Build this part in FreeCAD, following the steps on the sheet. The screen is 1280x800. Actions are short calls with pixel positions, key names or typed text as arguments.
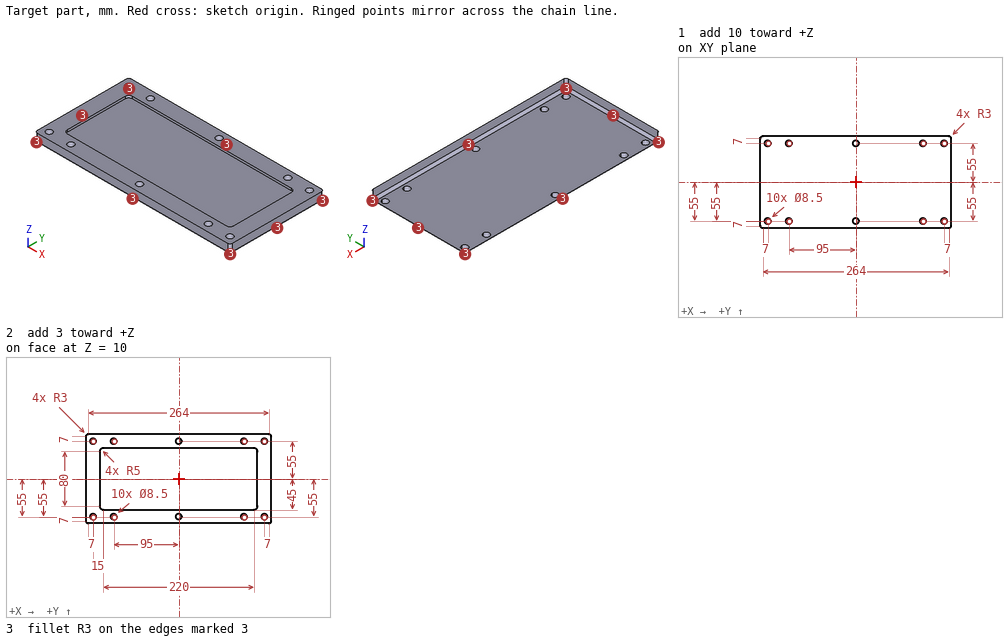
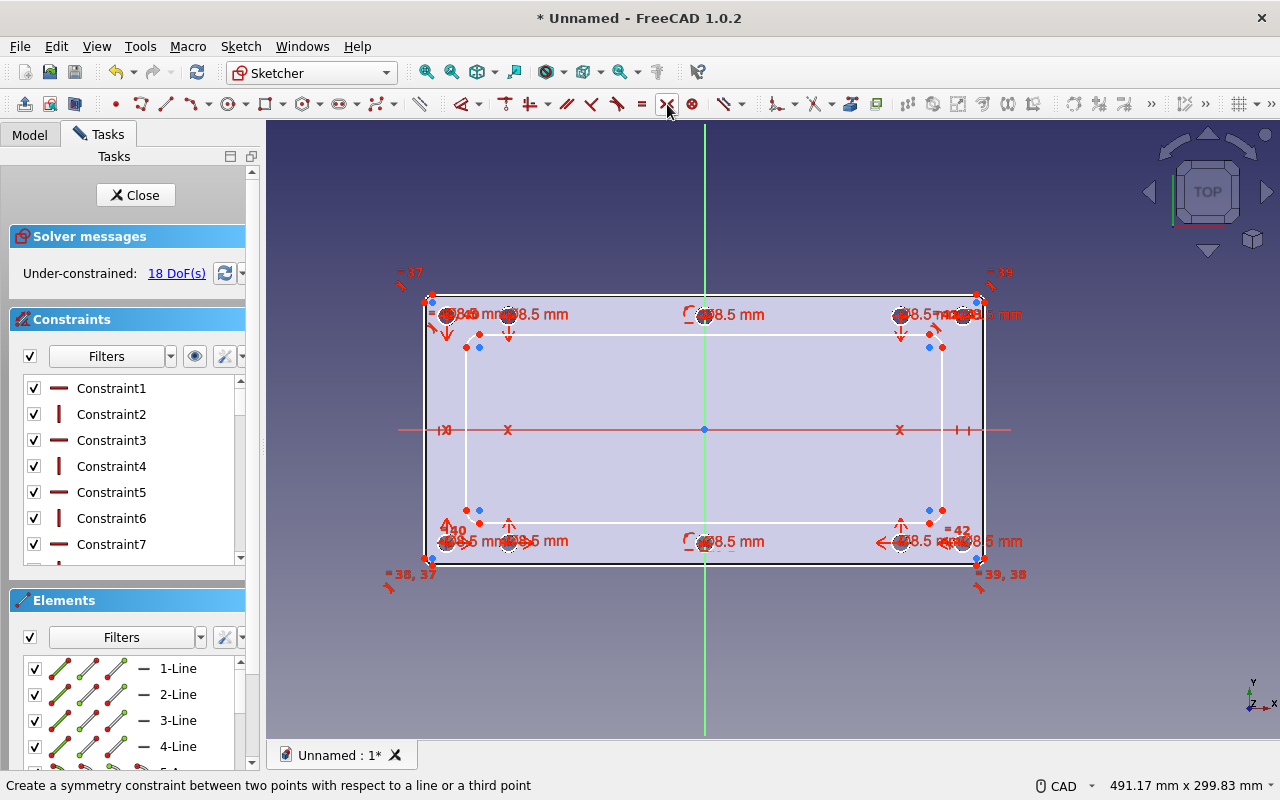
scroll(963, 543, up, 4)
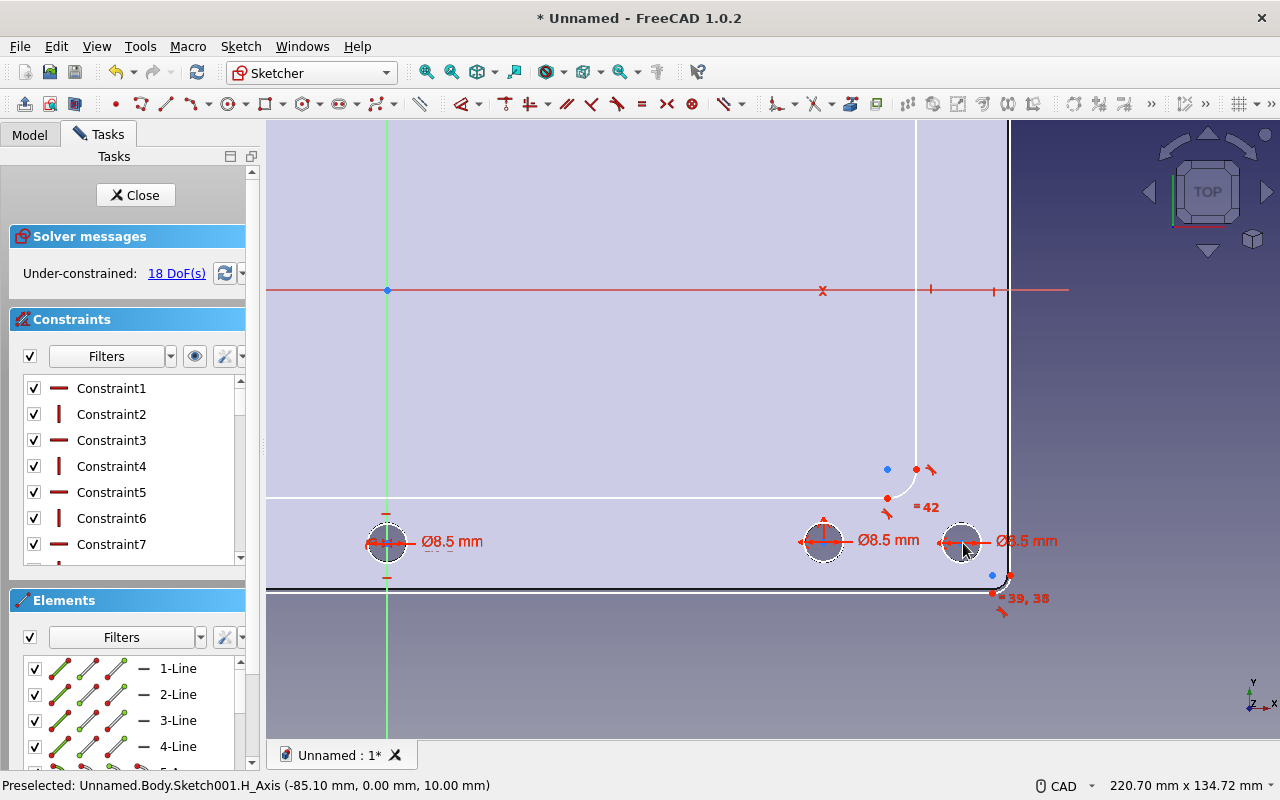
click(962, 543)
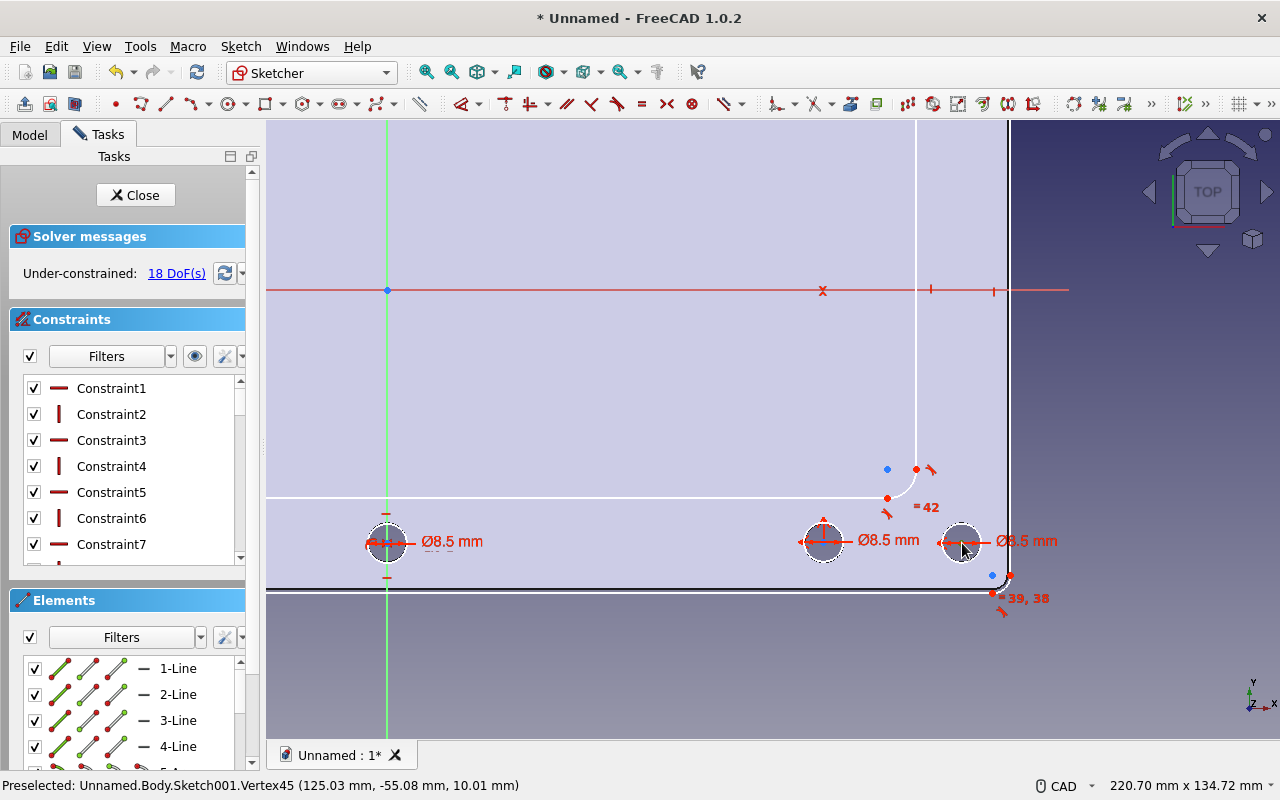
scroll(963, 543, down, 4)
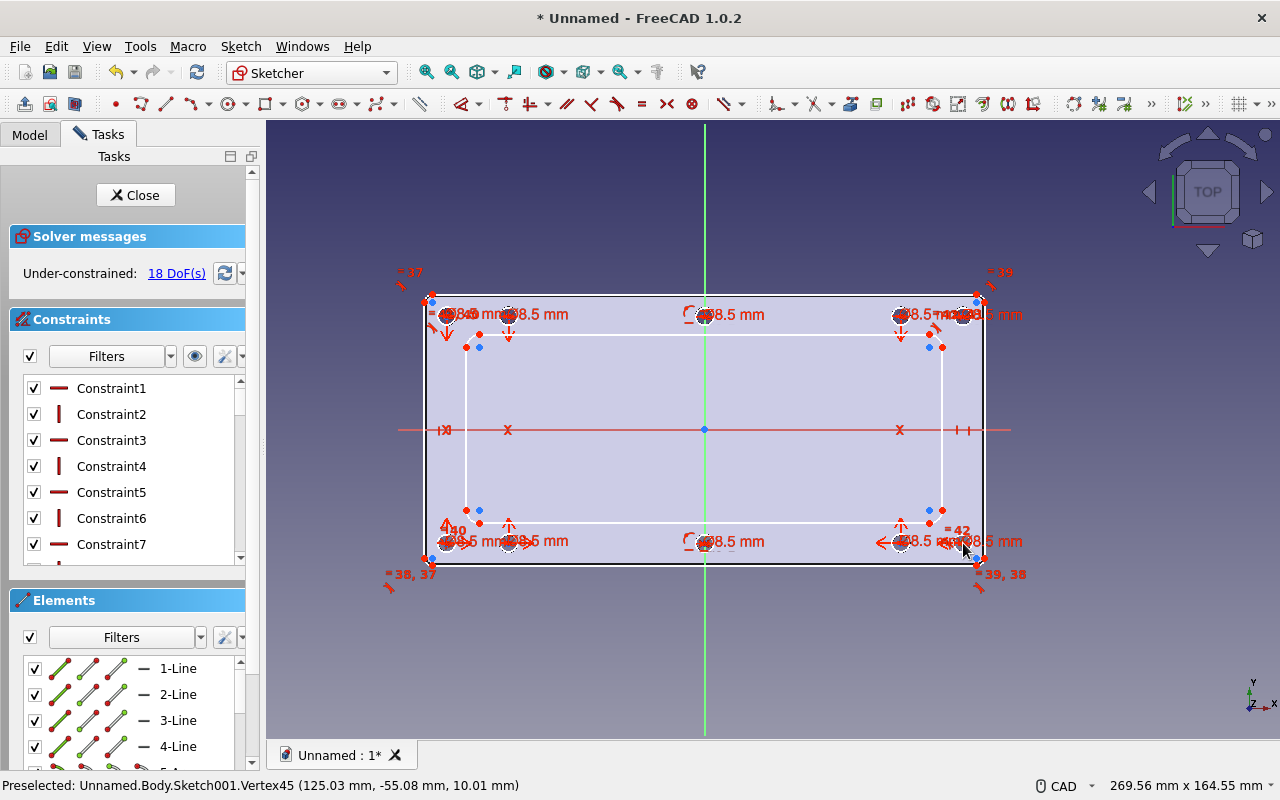
click(963, 317)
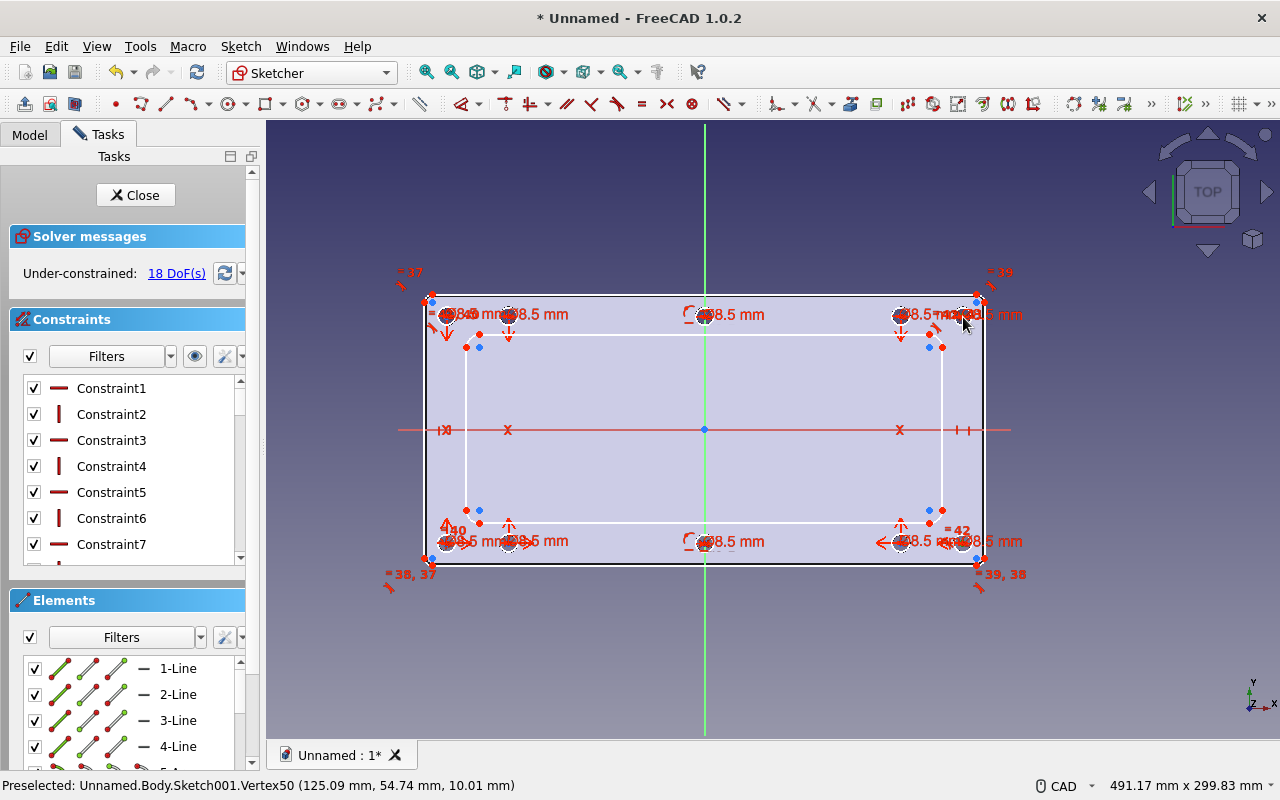
click(529, 430)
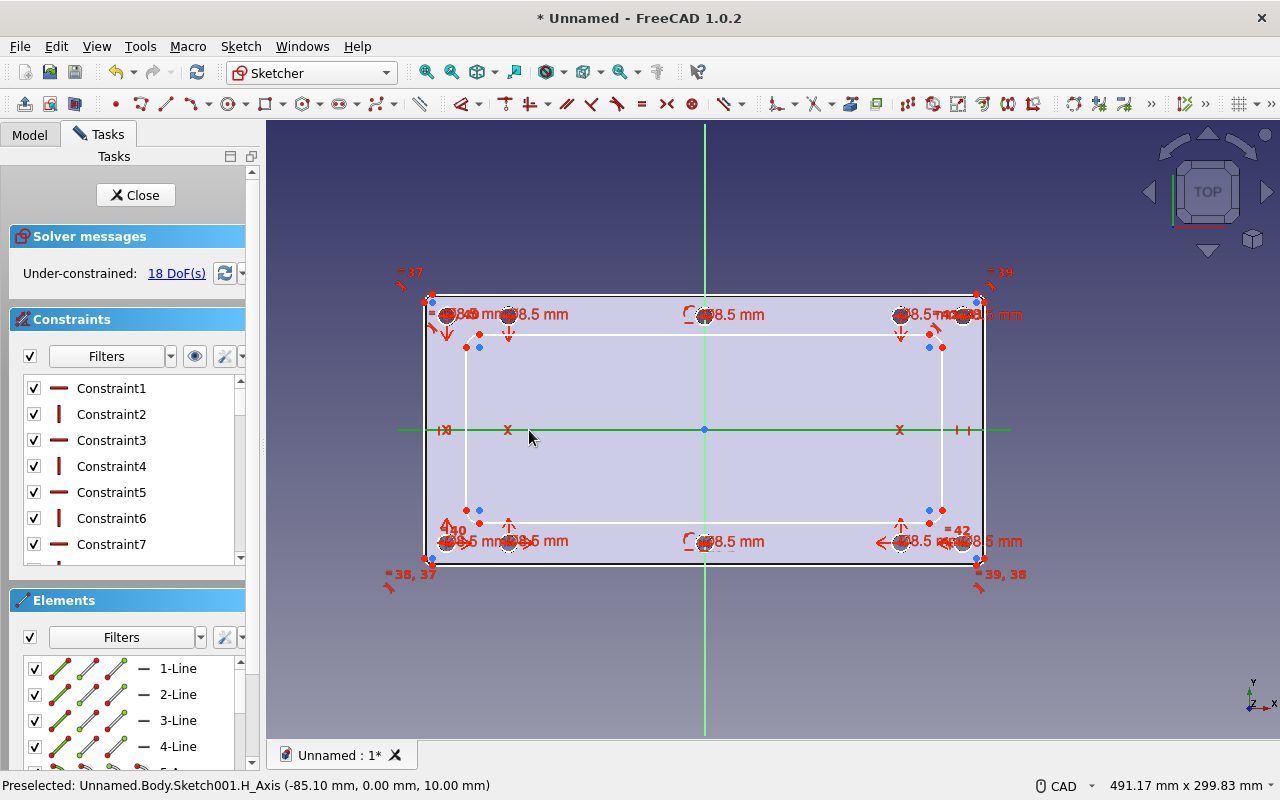
click(667, 104)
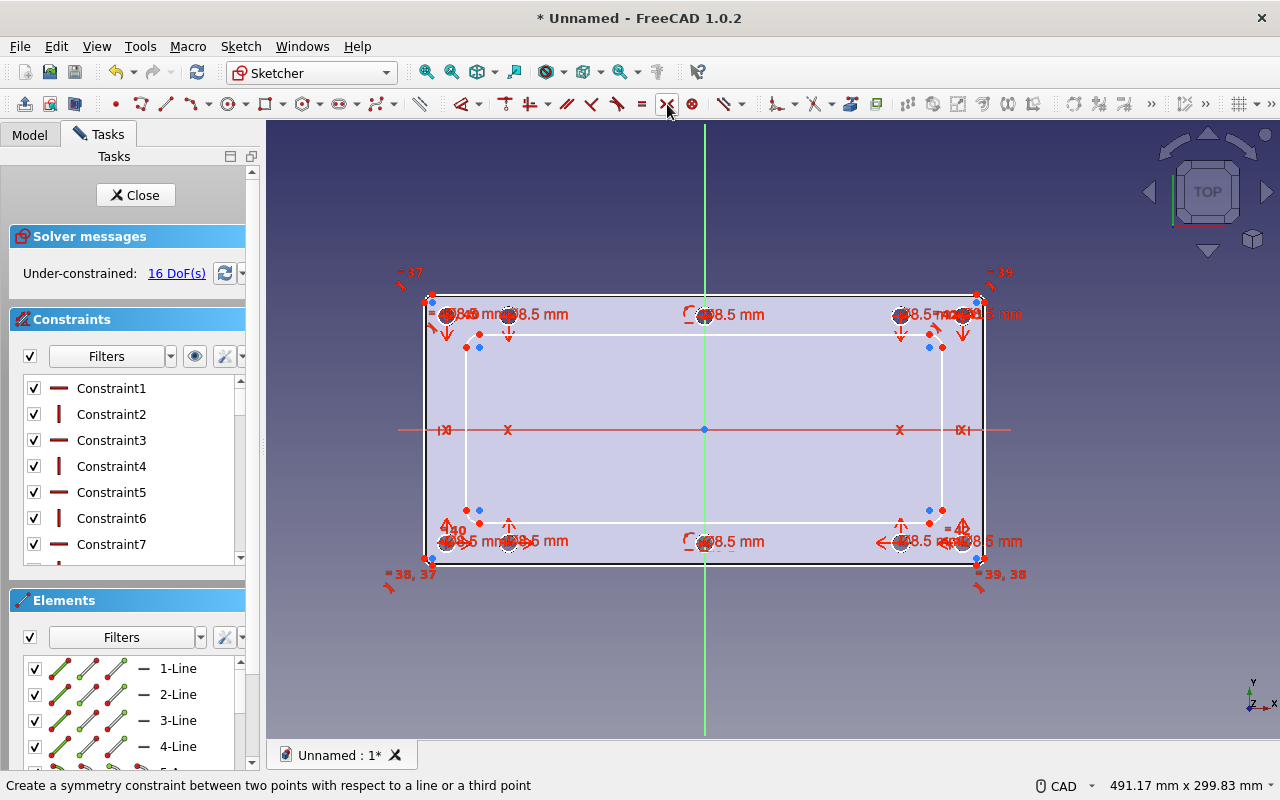
click(460, 104)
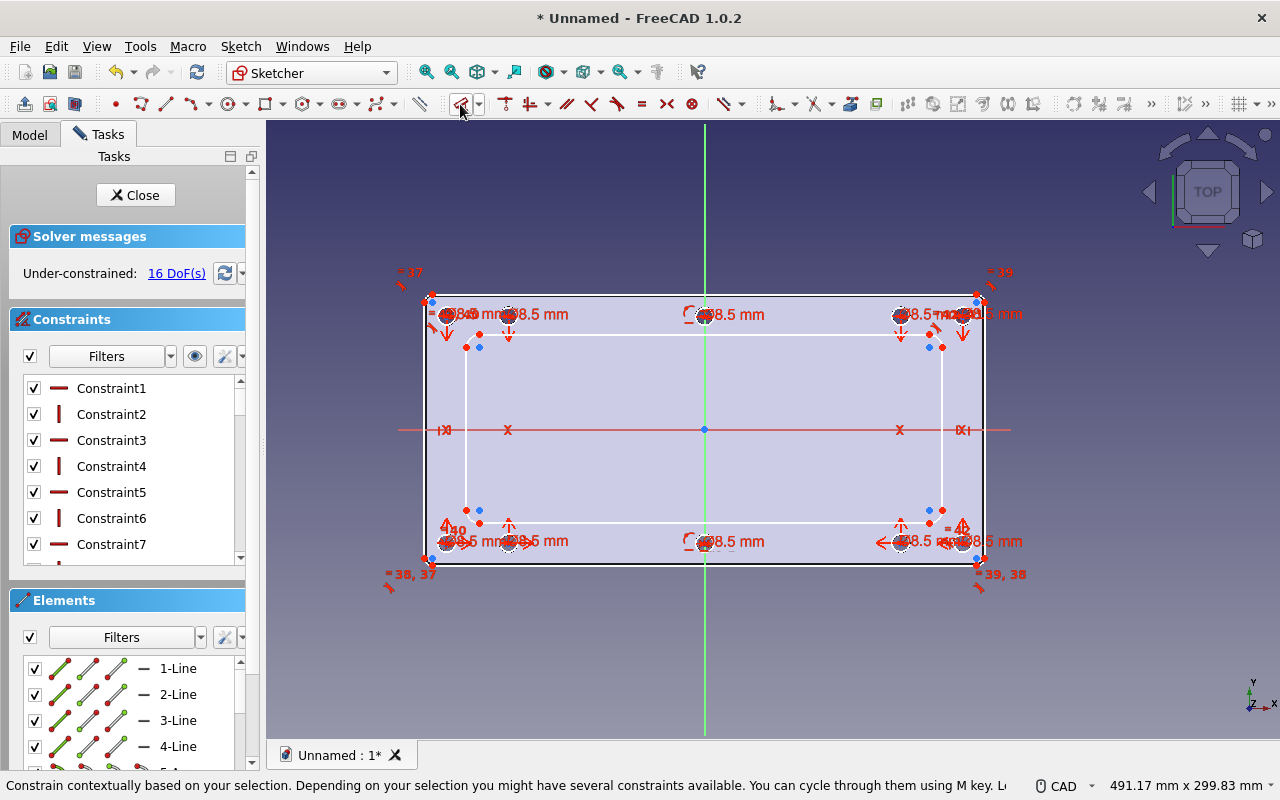
scroll(427, 297, up, 10)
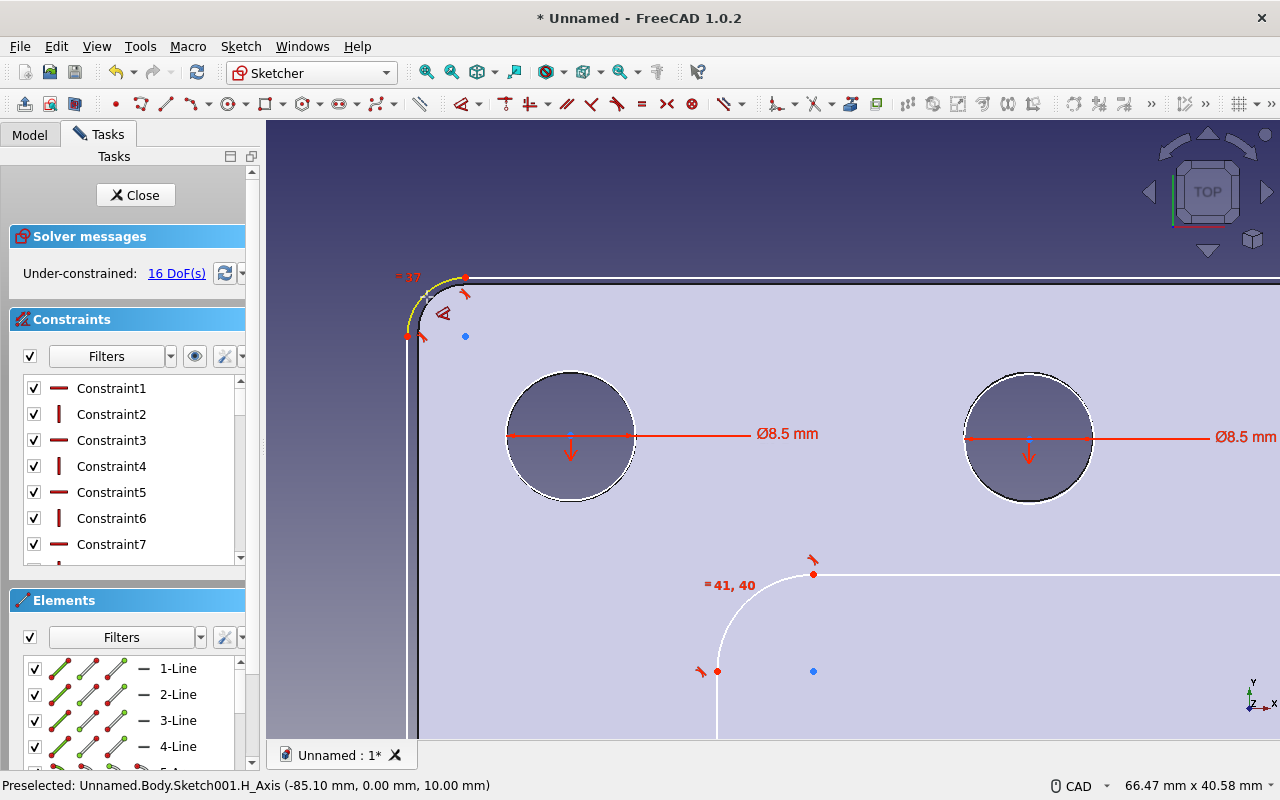
click(425, 295)
click(402, 272)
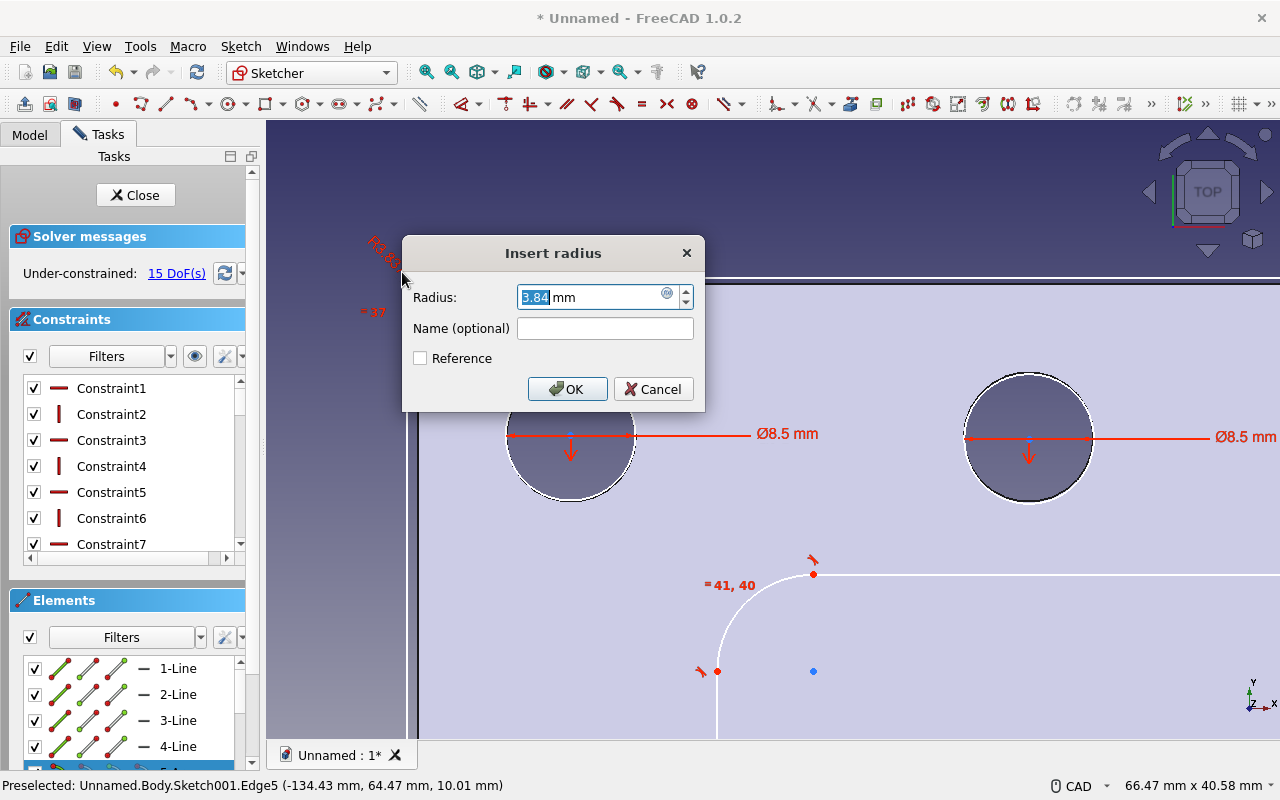
text(3)
key(Return)